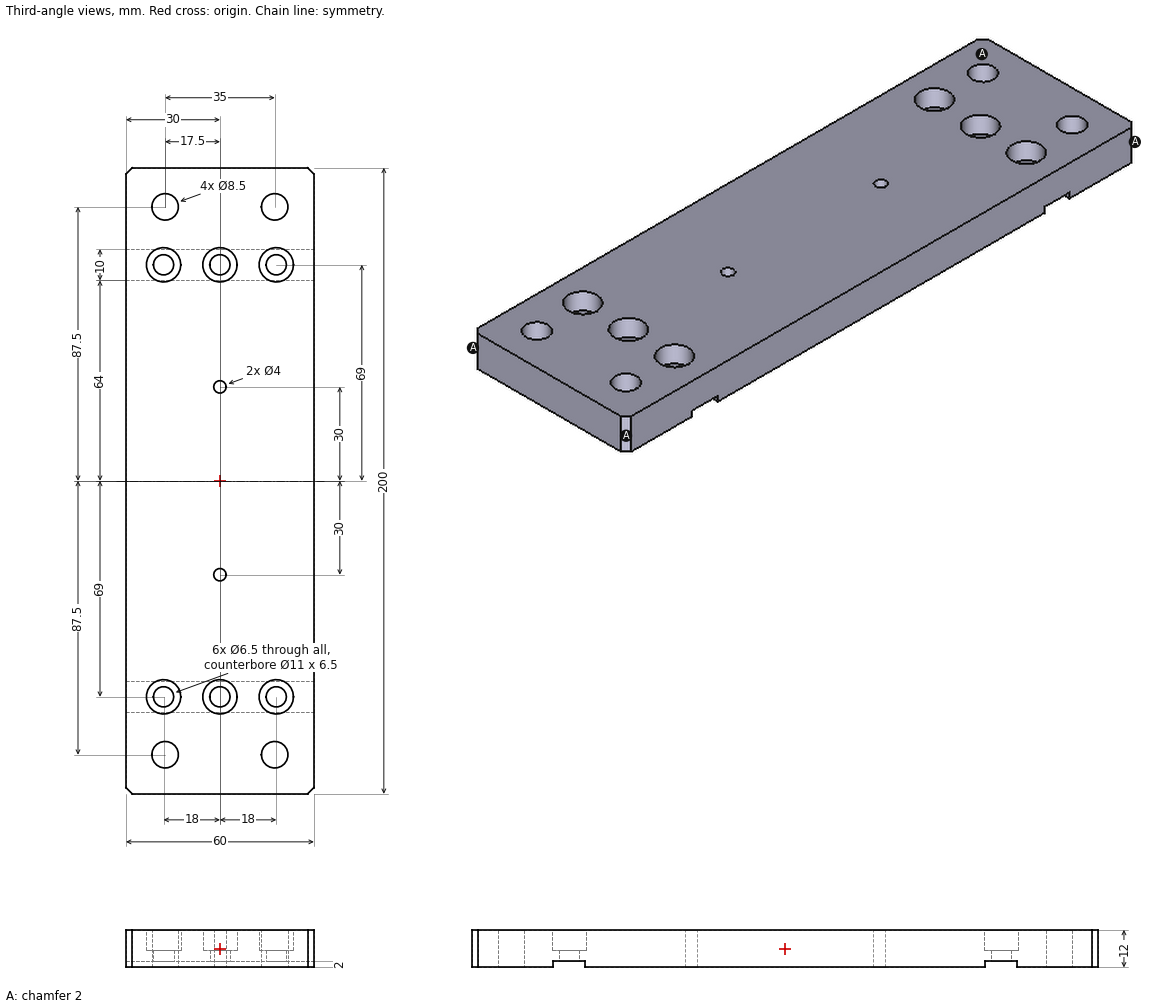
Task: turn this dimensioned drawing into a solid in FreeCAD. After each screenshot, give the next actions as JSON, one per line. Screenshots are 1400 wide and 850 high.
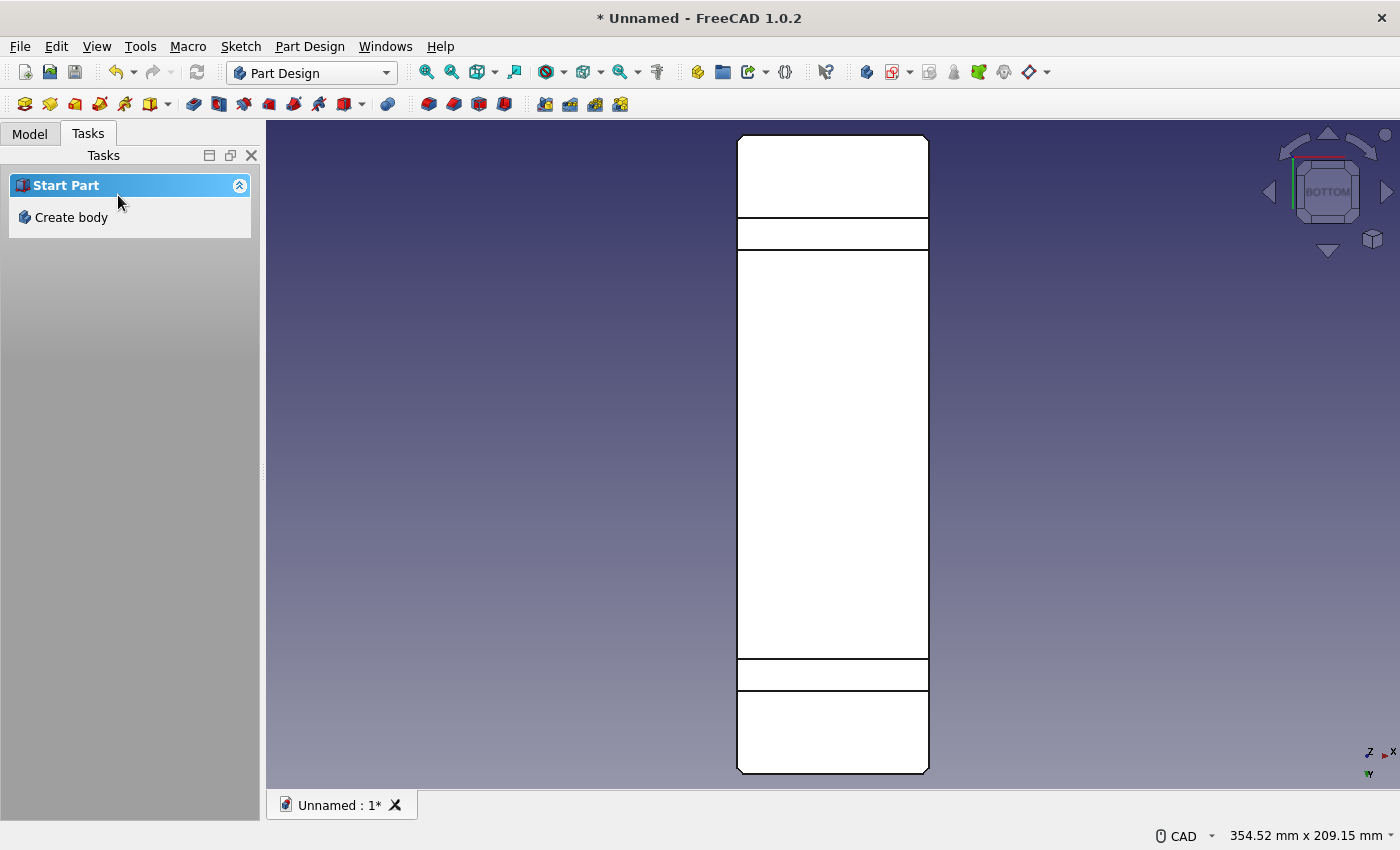
{"action": "key", "text": "0"}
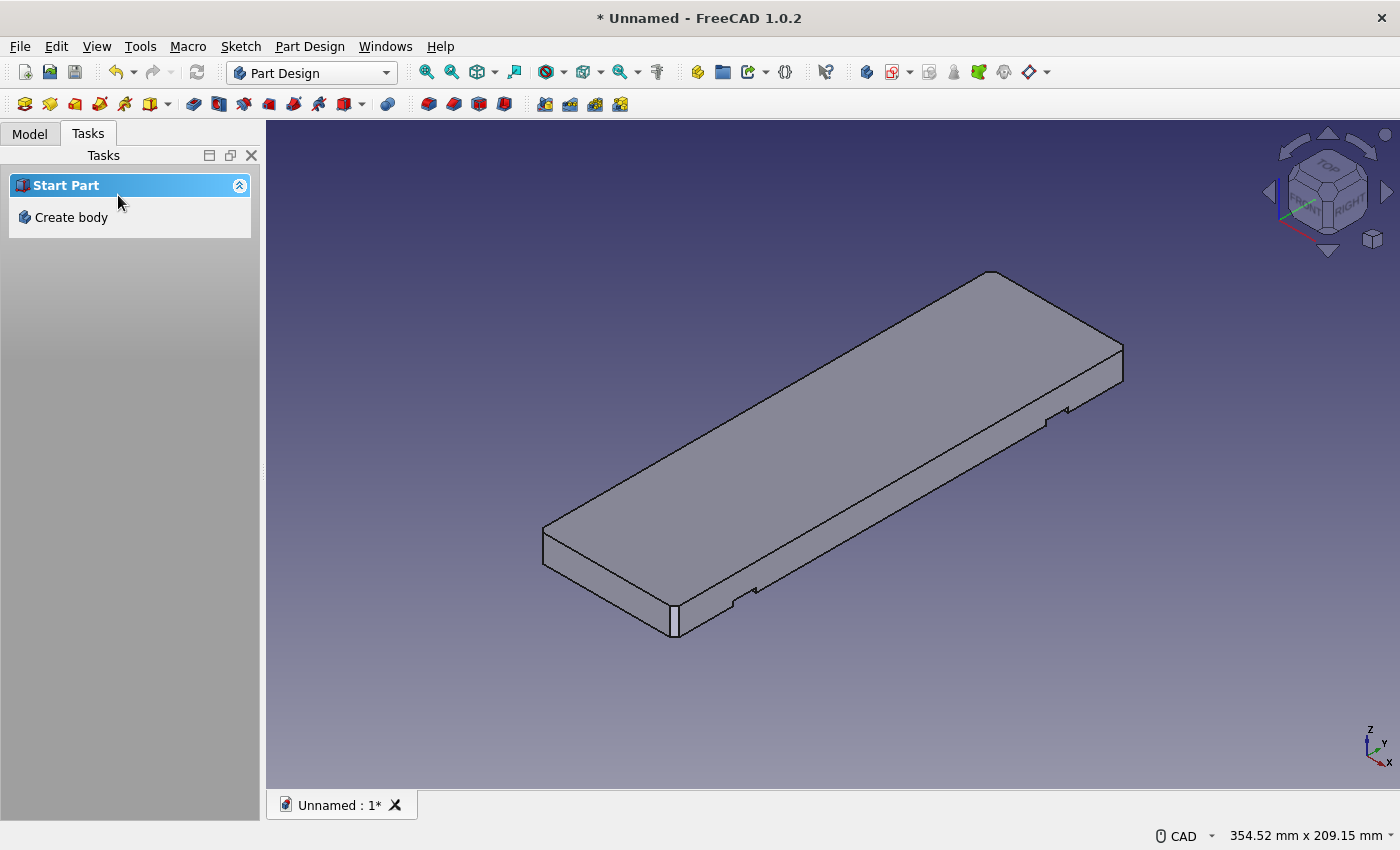
{"action": "left_click", "coordinate": [962, 363]}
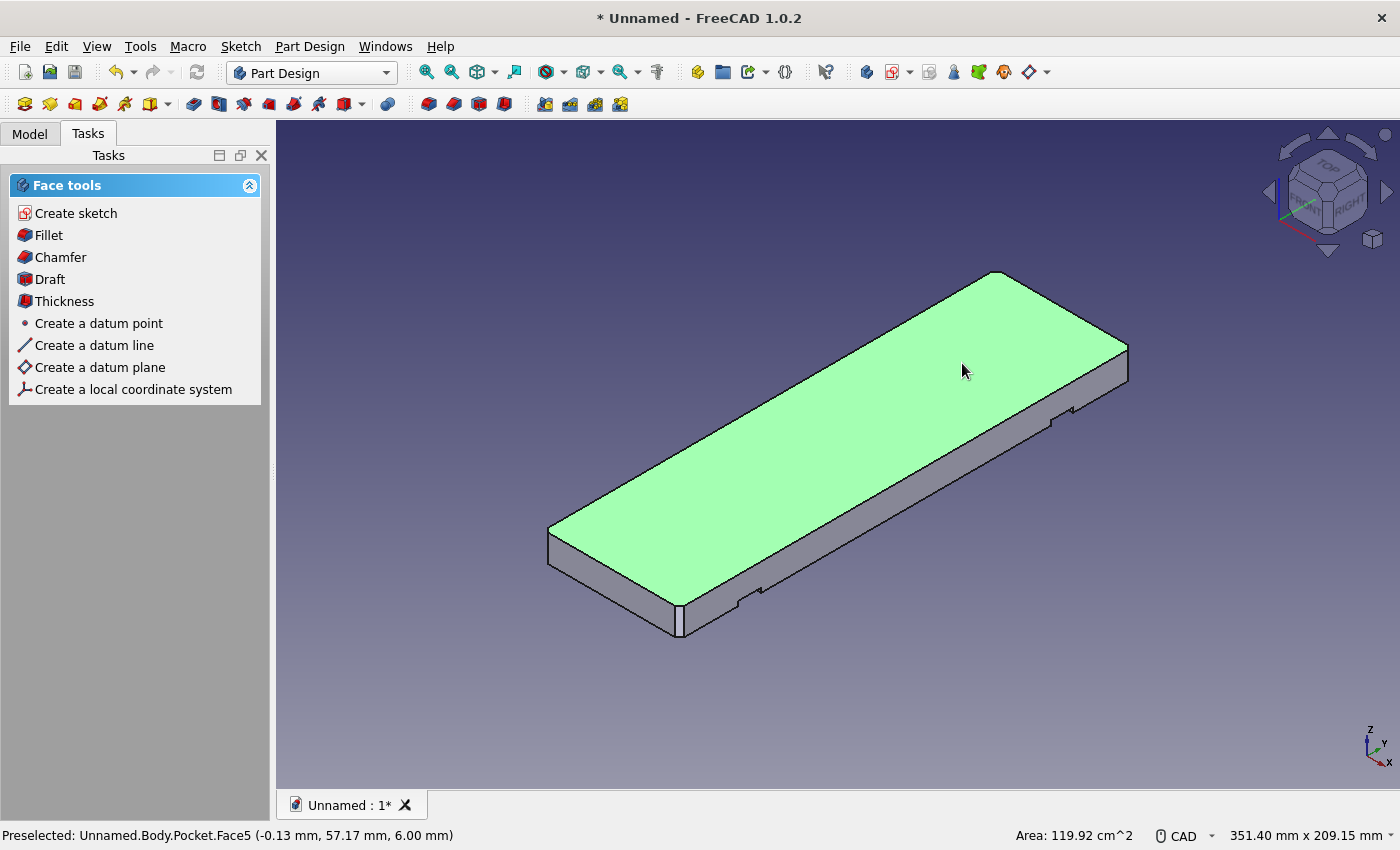
{"action": "left_click", "coordinate": [892, 72]}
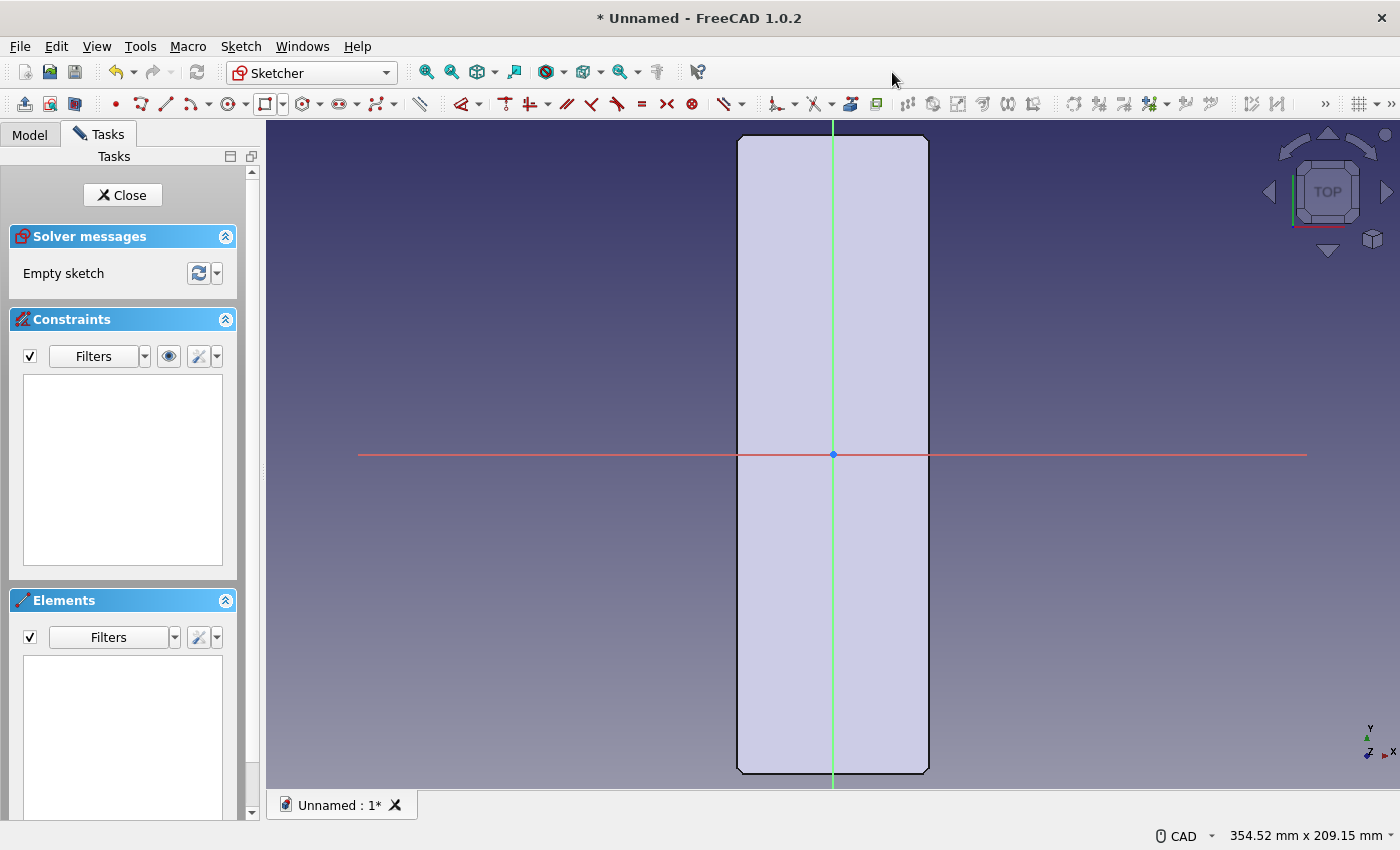
{"action": "left_click", "coordinate": [228, 104]}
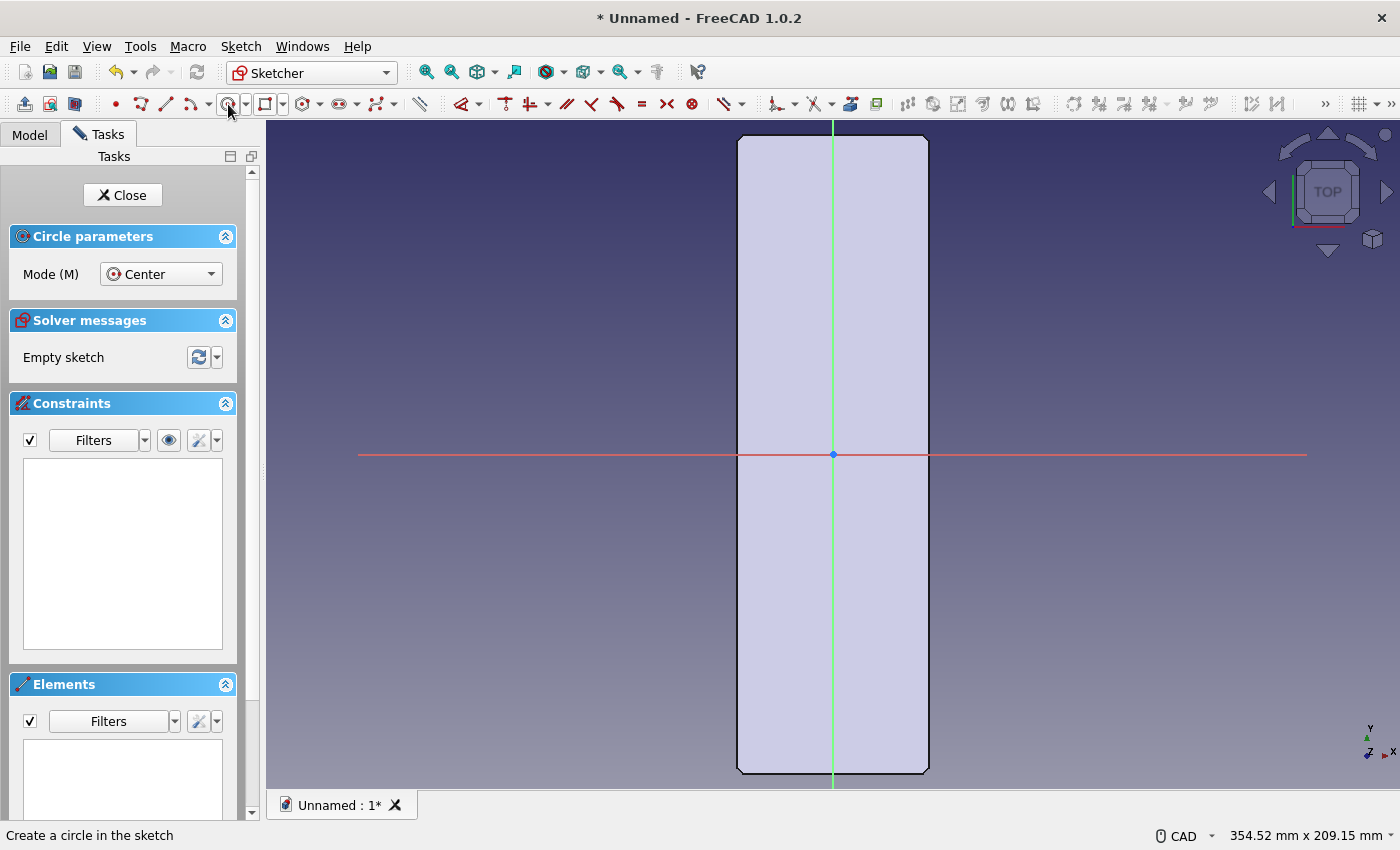
{"action": "scroll", "coordinate": [775, 675], "scroll_direction": "up", "scroll_amount": 4}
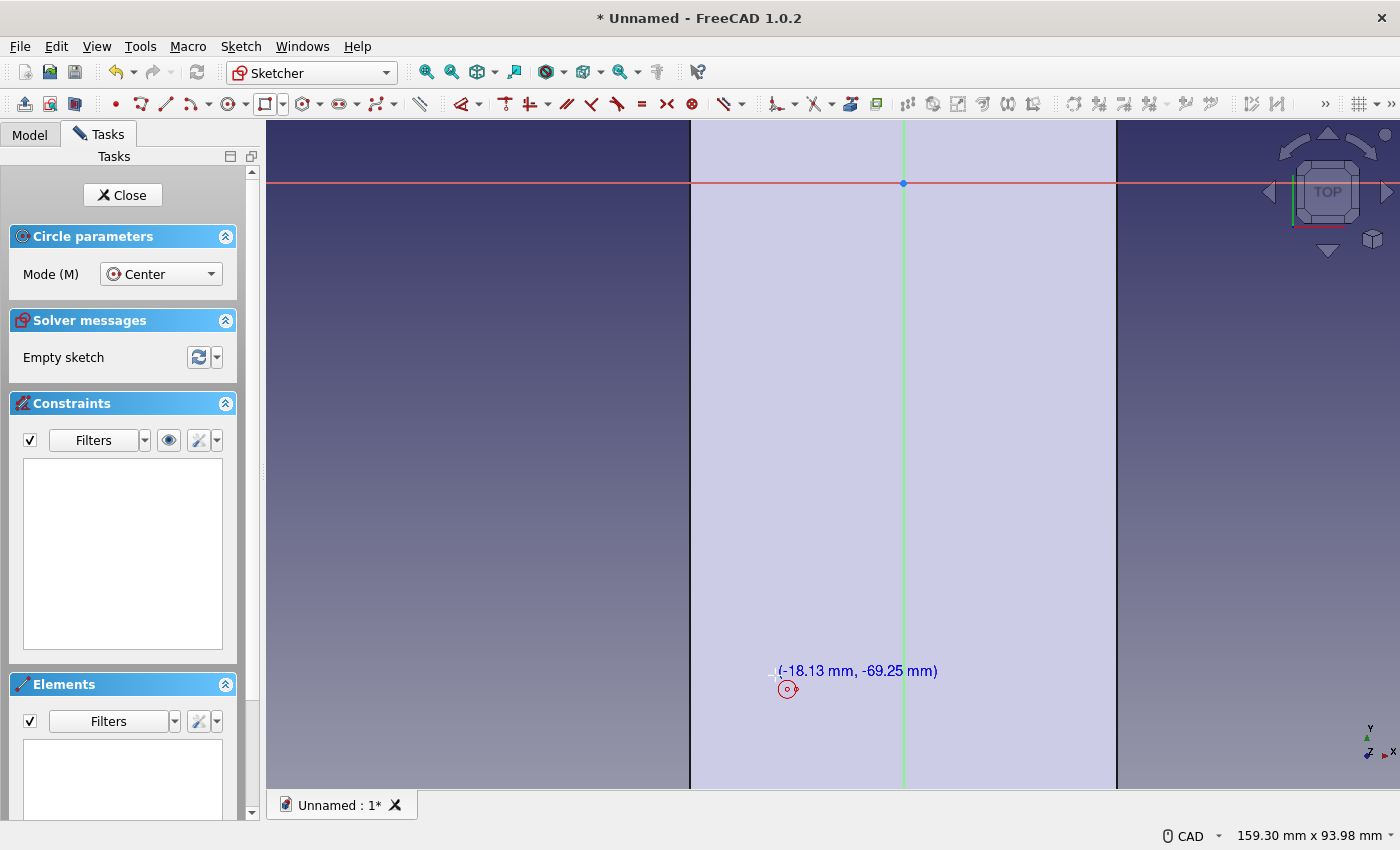
{"action": "left_click", "coordinate": [775, 674]}
{"action": "left_click", "coordinate": [792, 658]}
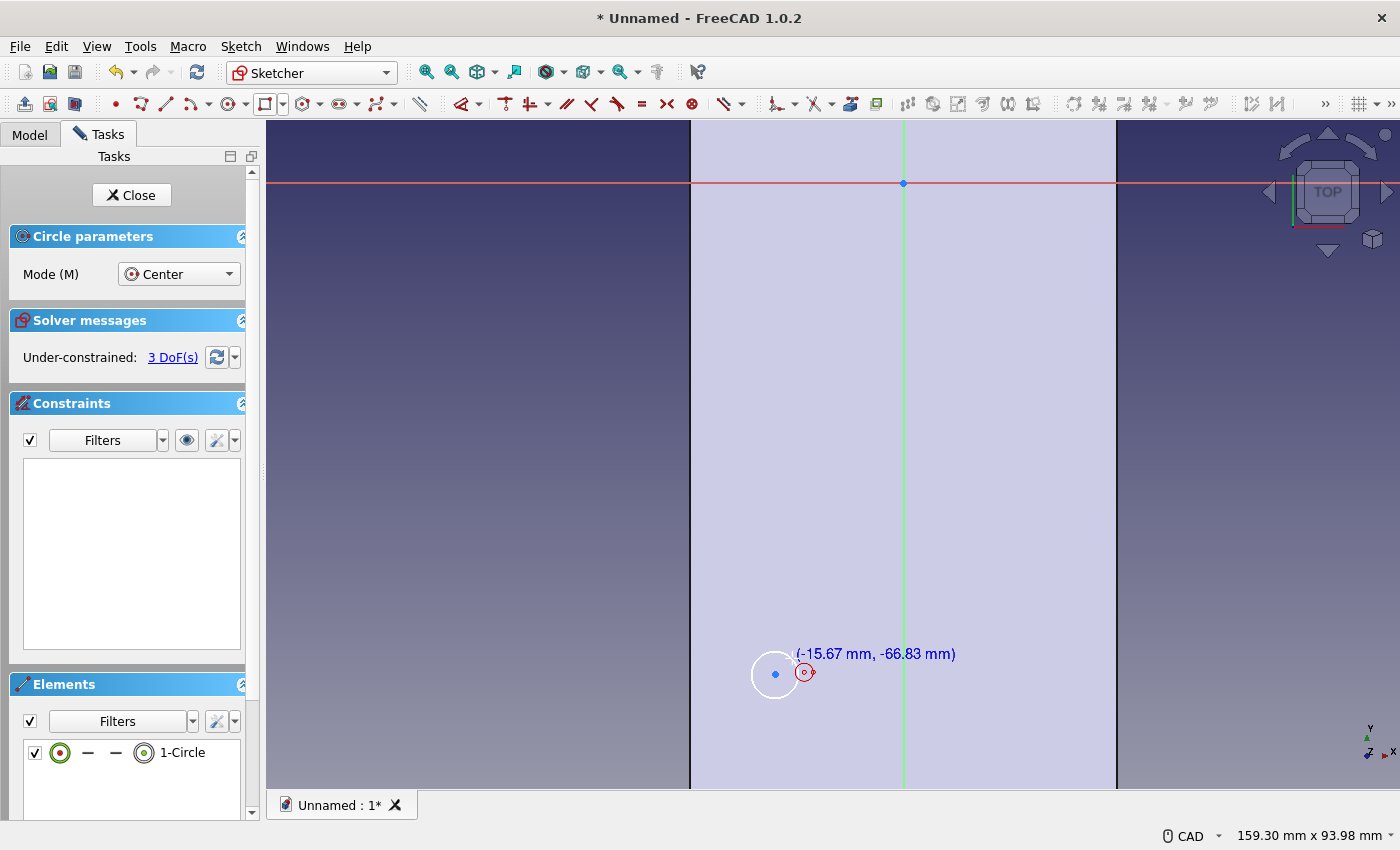
{"action": "left_click", "coordinate": [904, 674]}
{"action": "left_click", "coordinate": [920, 658]}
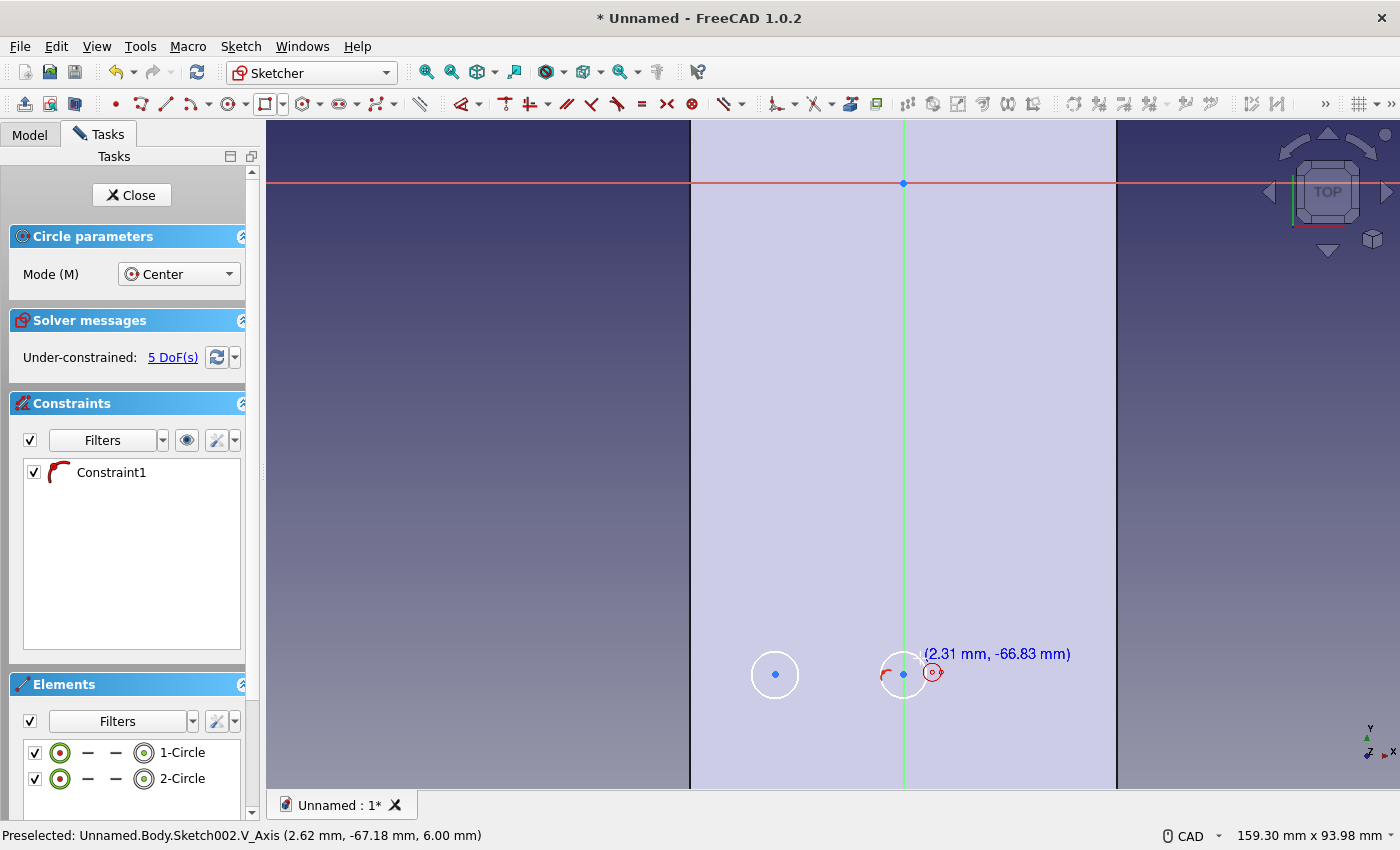
{"action": "left_click", "coordinate": [1032, 674]}
{"action": "left_click", "coordinate": [1048, 658]}